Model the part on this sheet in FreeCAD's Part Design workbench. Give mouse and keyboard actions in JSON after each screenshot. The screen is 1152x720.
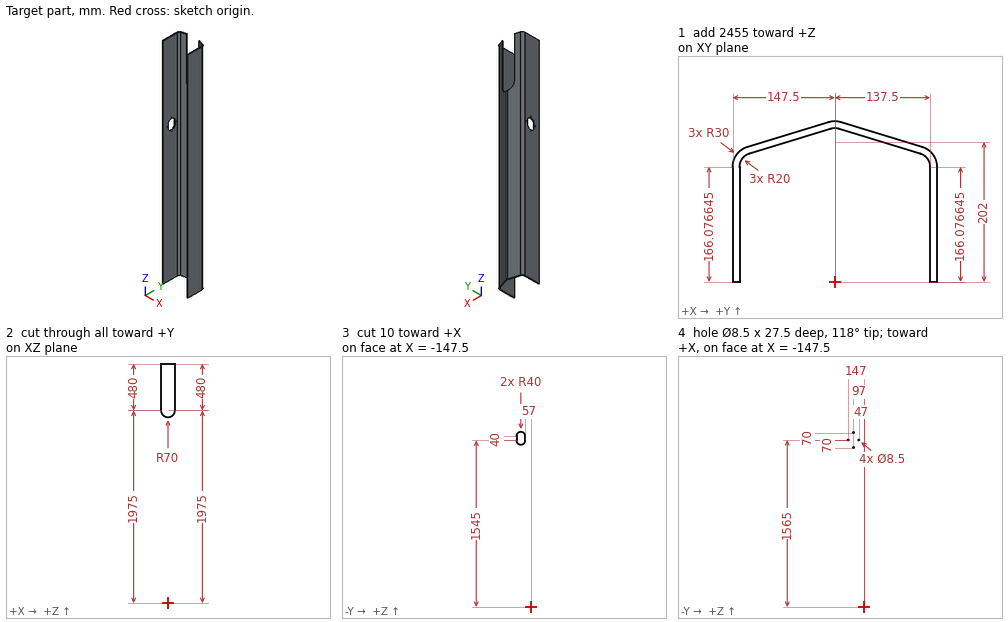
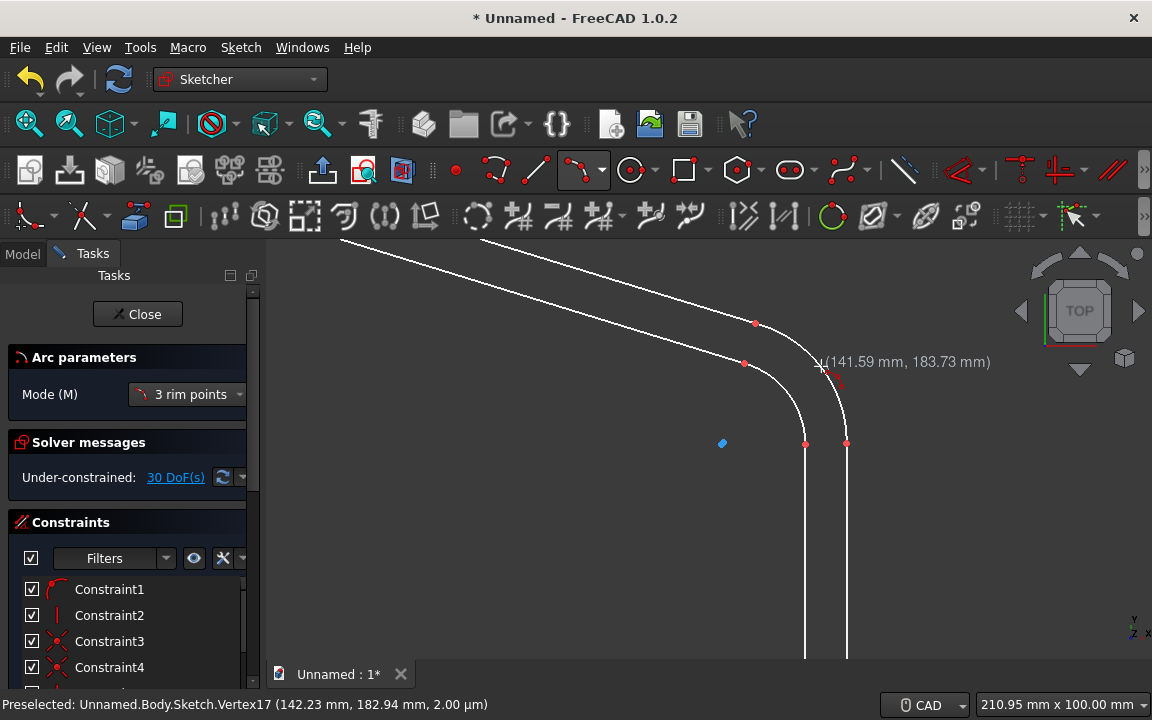
{"action": "scroll", "coordinate": [776, 383], "scroll_direction": "down", "scroll_amount": 7}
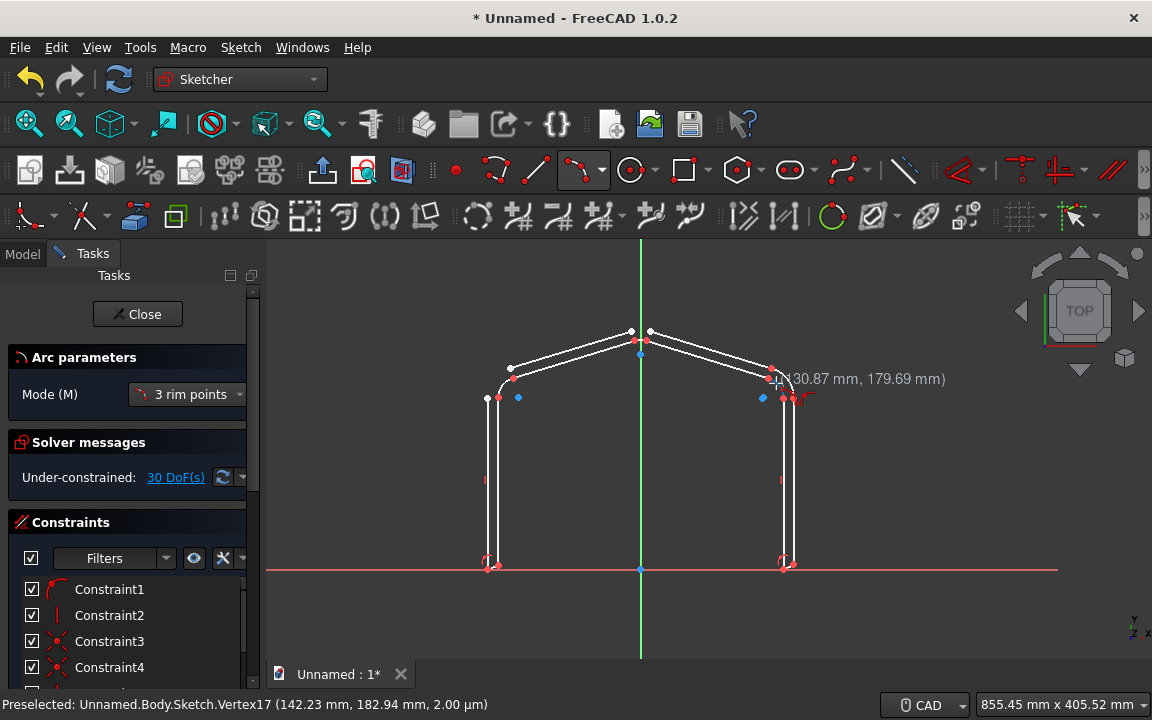
{"action": "scroll", "coordinate": [650, 331], "scroll_direction": "up", "scroll_amount": 3}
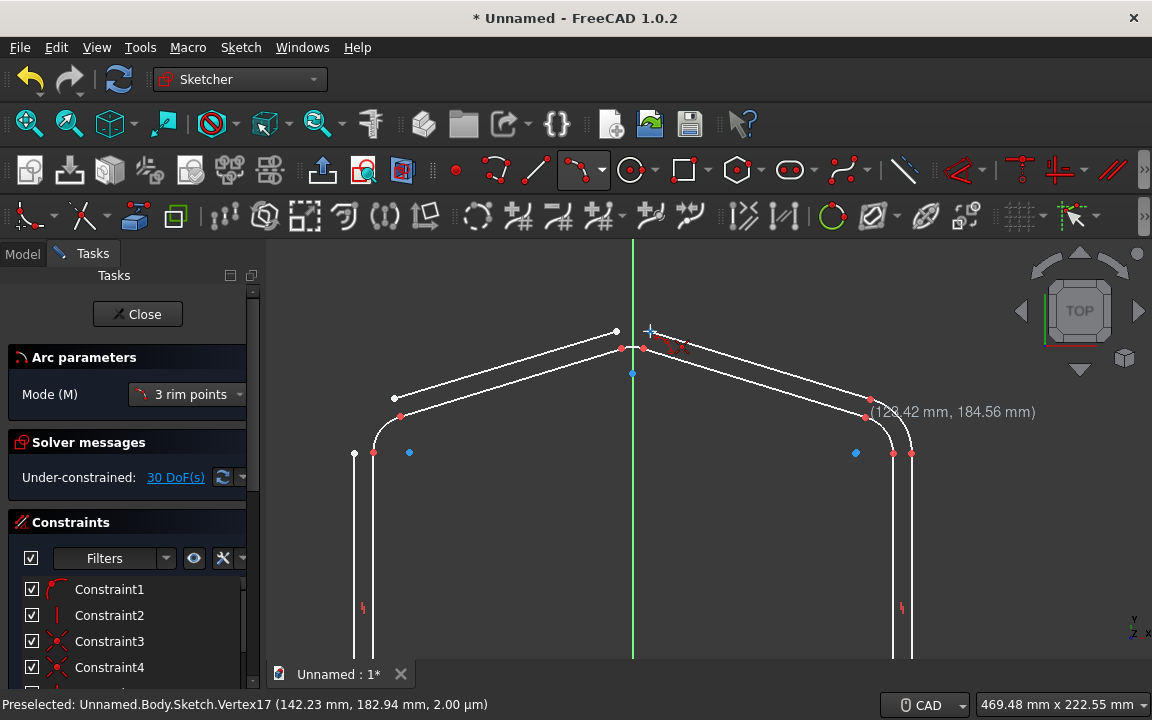
{"action": "left_click", "coordinate": [650, 332]}
{"action": "left_click", "coordinate": [616, 332]}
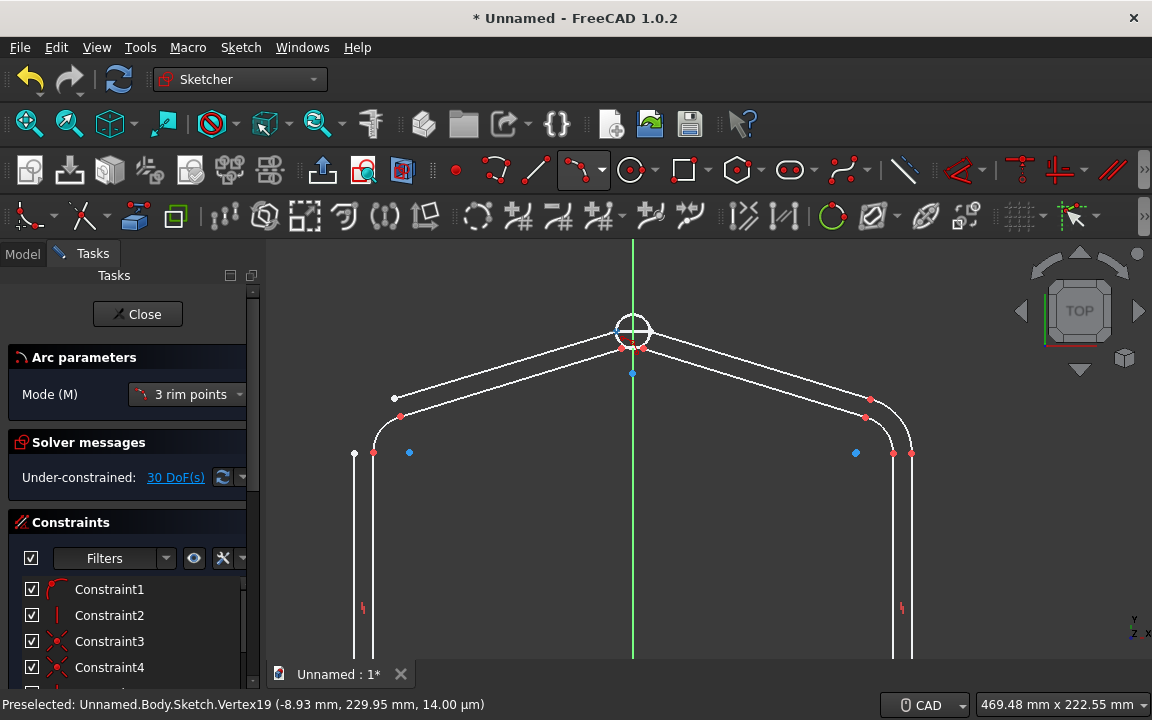
{"action": "scroll", "coordinate": [636, 328], "scroll_direction": "up", "scroll_amount": 10}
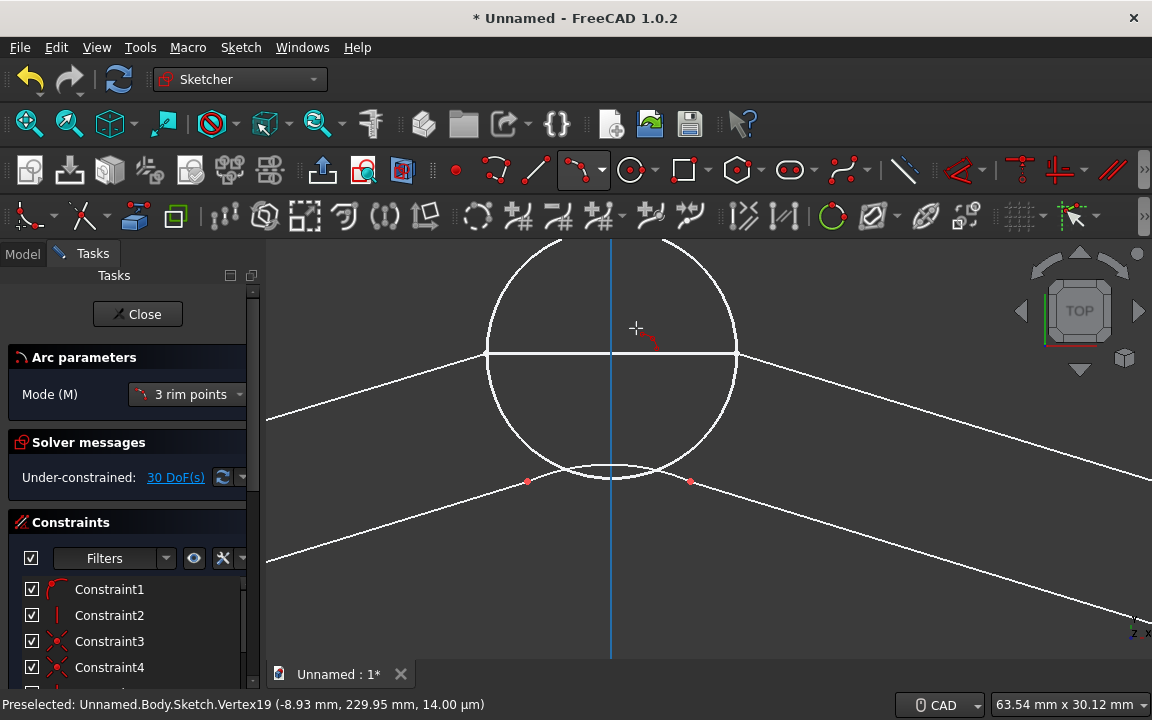
{"action": "left_click", "coordinate": [636, 326]}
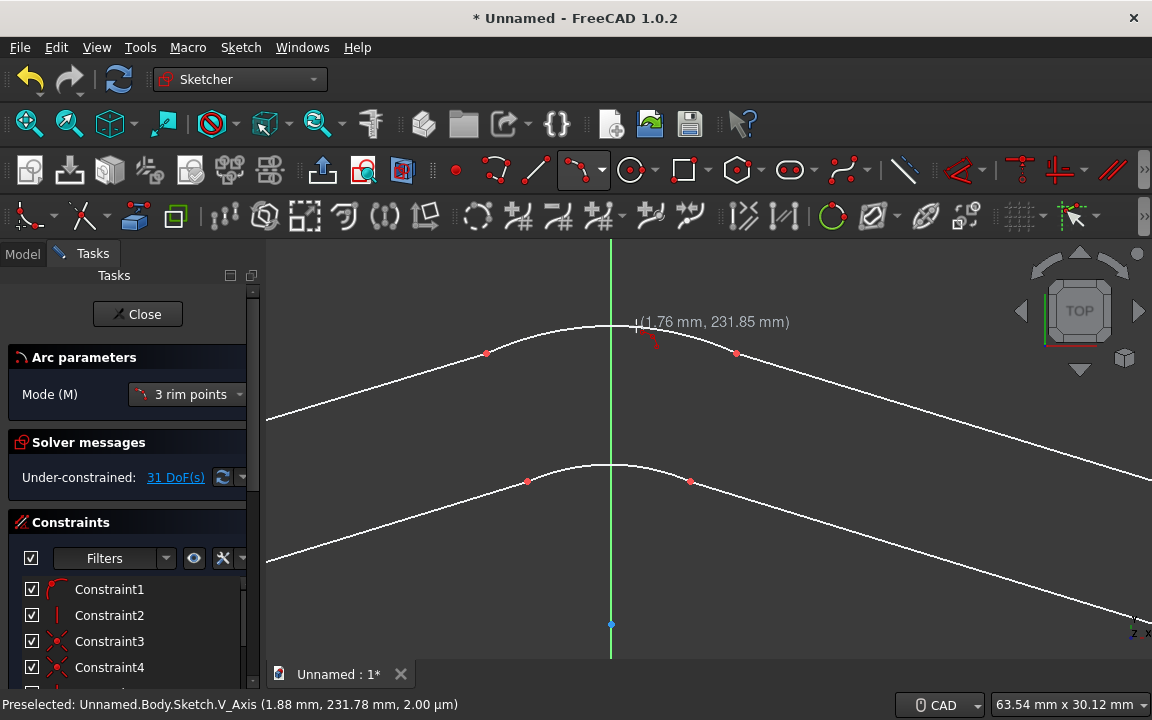
{"action": "scroll", "coordinate": [643, 329], "scroll_direction": "down", "scroll_amount": 13}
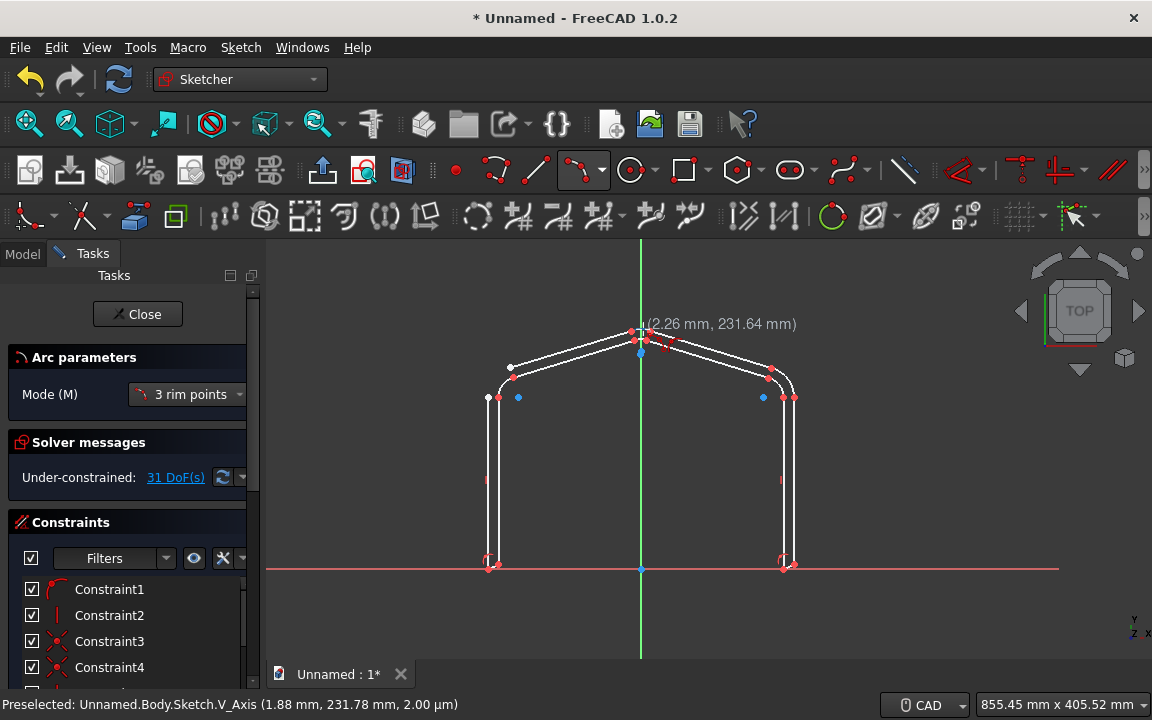
{"action": "scroll", "coordinate": [510, 367], "scroll_direction": "up", "scroll_amount": 3}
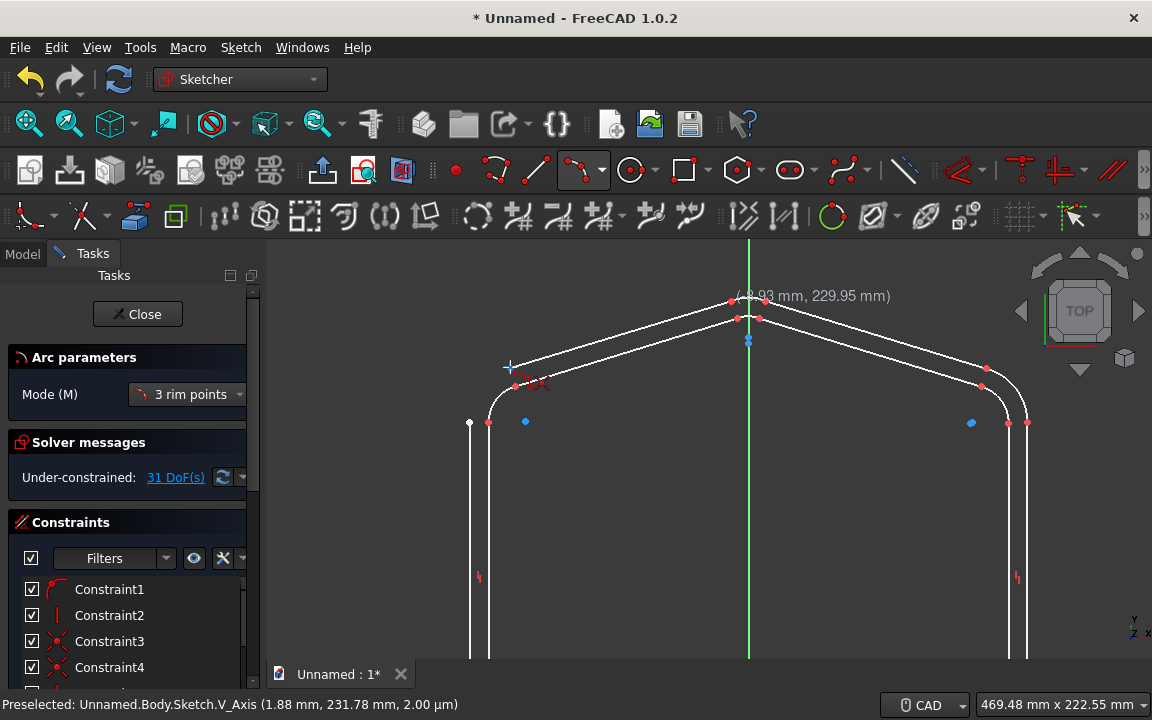
{"action": "left_click", "coordinate": [510, 368]}
{"action": "left_click", "coordinate": [470, 423]}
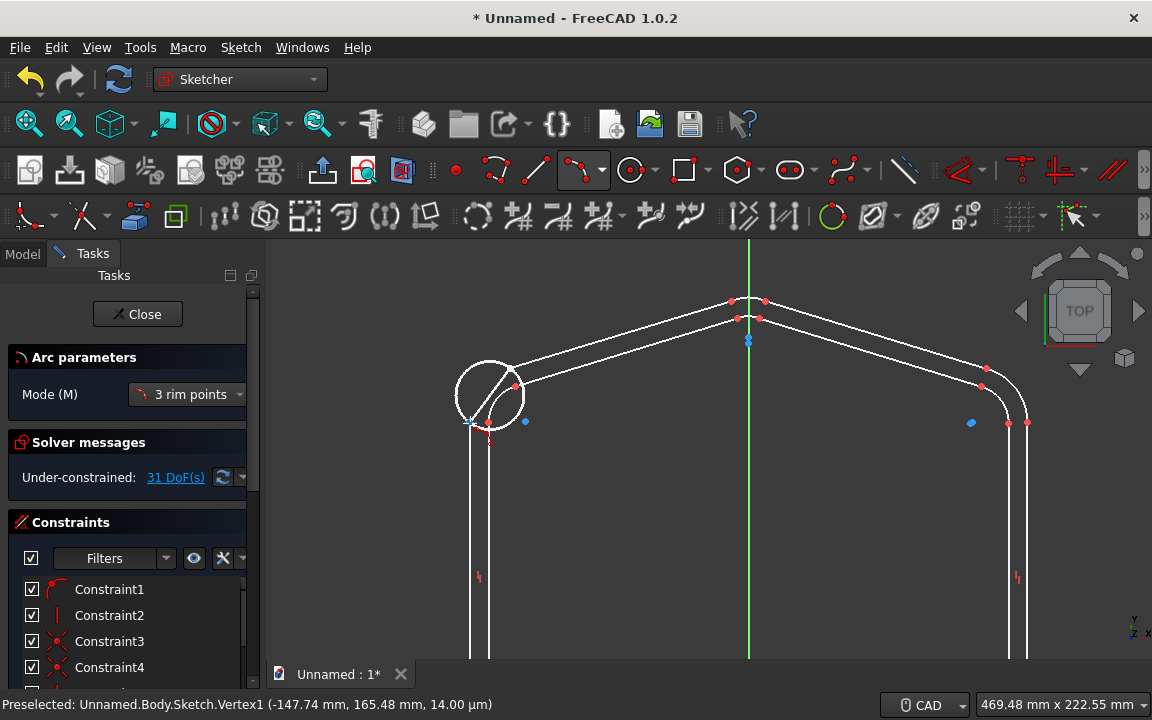
{"action": "scroll", "coordinate": [481, 388], "scroll_direction": "up", "scroll_amount": 2}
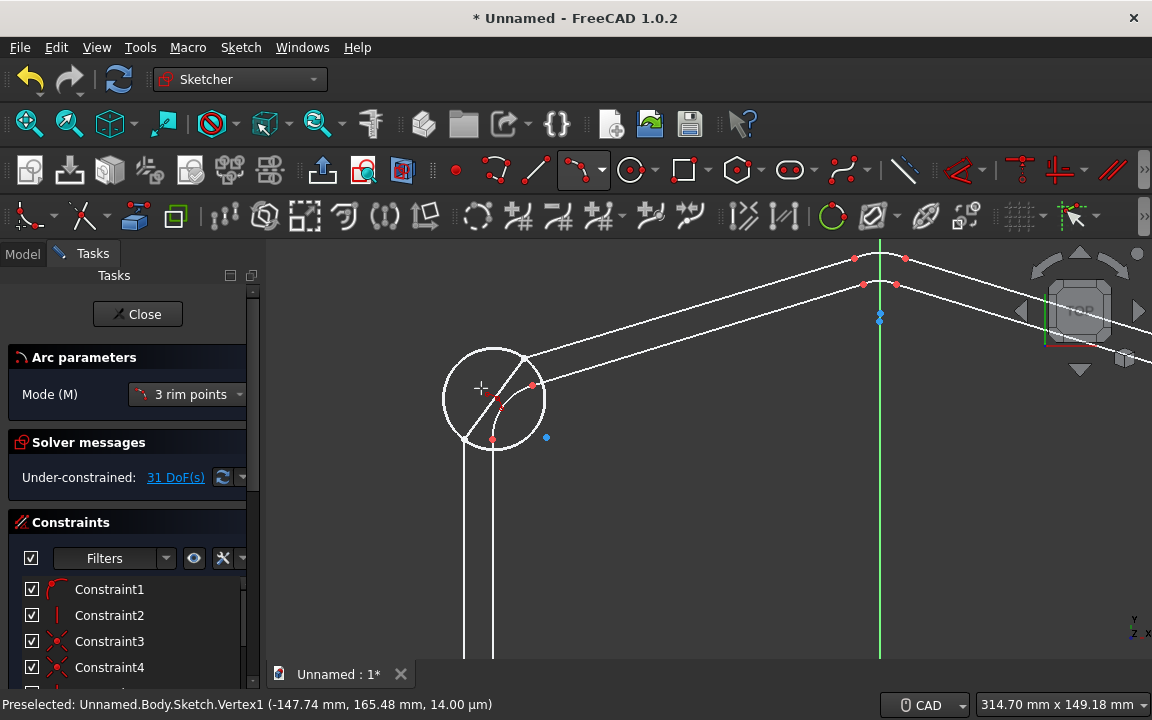
{"action": "left_click", "coordinate": [481, 388]}
{"action": "key", "text": "Escape"}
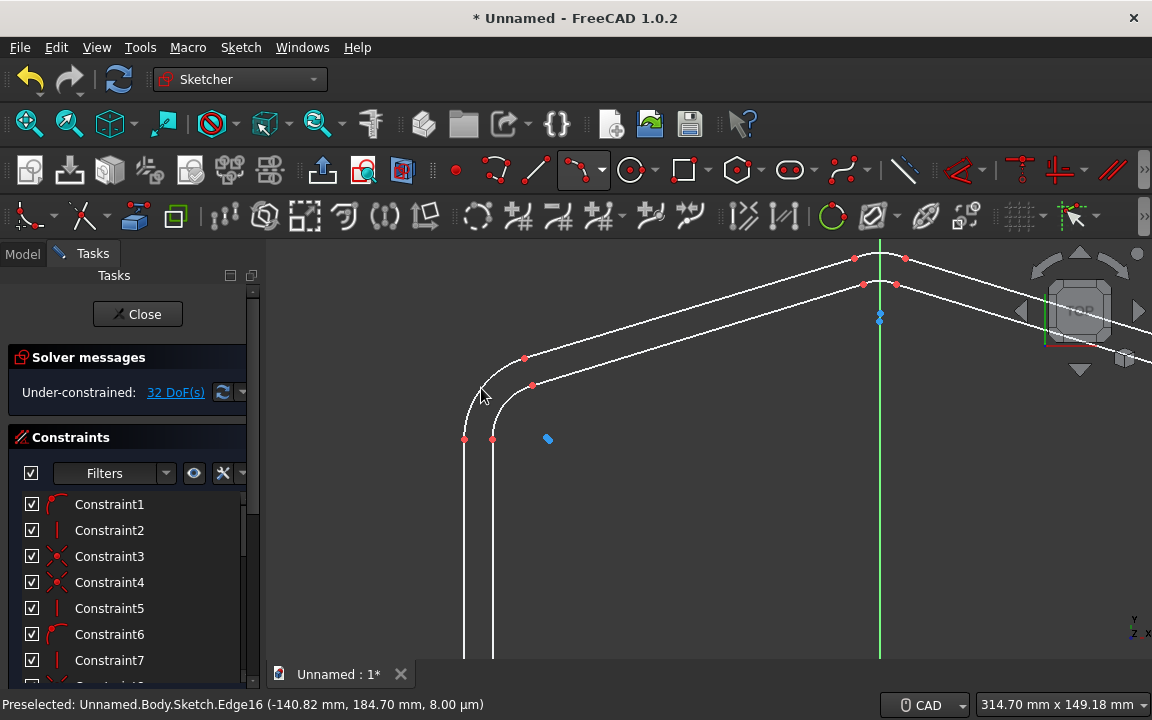
{"action": "left_click", "coordinate": [464, 580]}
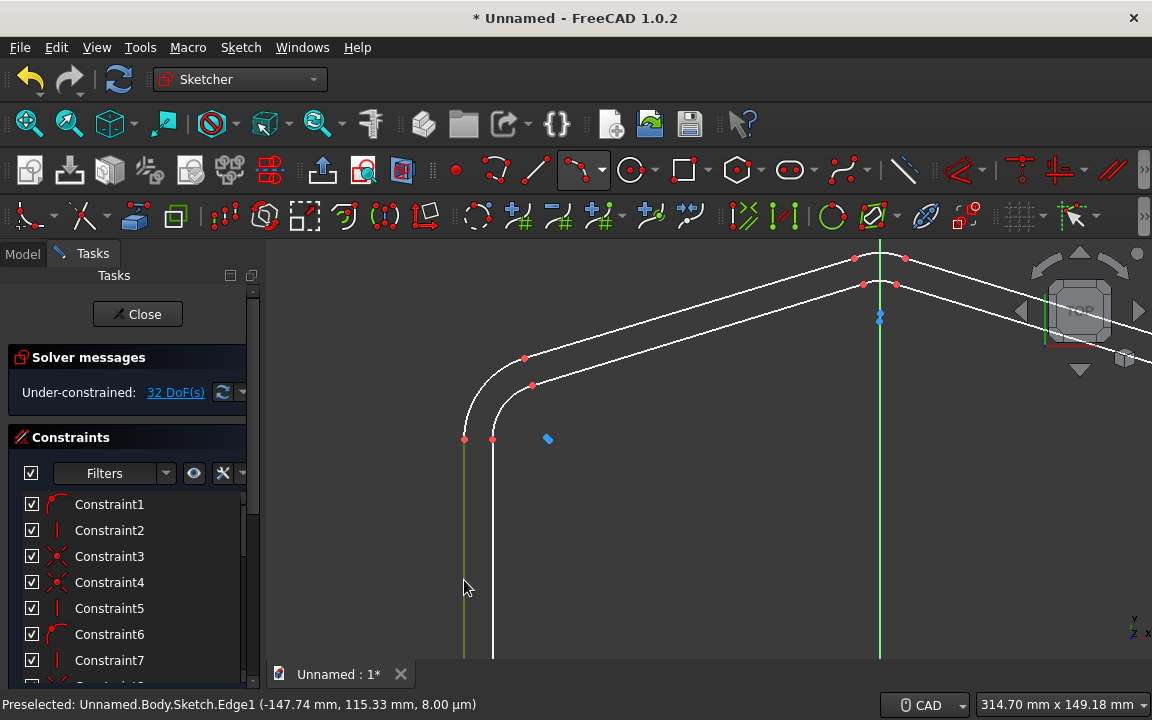
{"action": "left_click", "coordinate": [496, 373]}